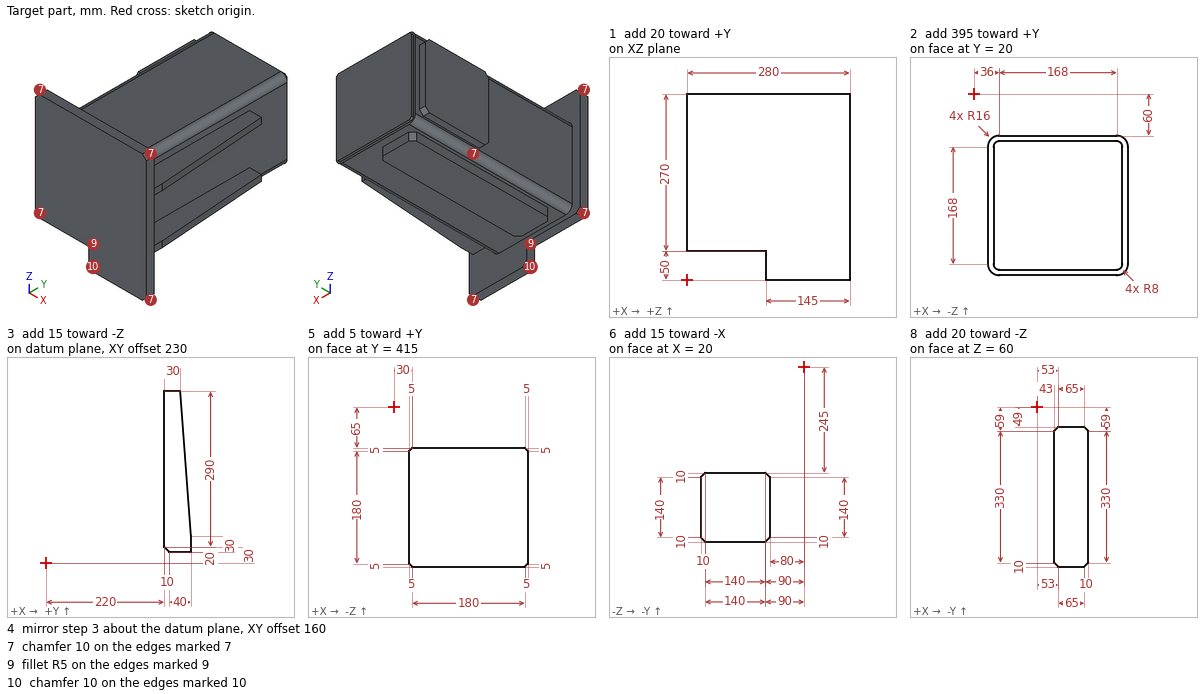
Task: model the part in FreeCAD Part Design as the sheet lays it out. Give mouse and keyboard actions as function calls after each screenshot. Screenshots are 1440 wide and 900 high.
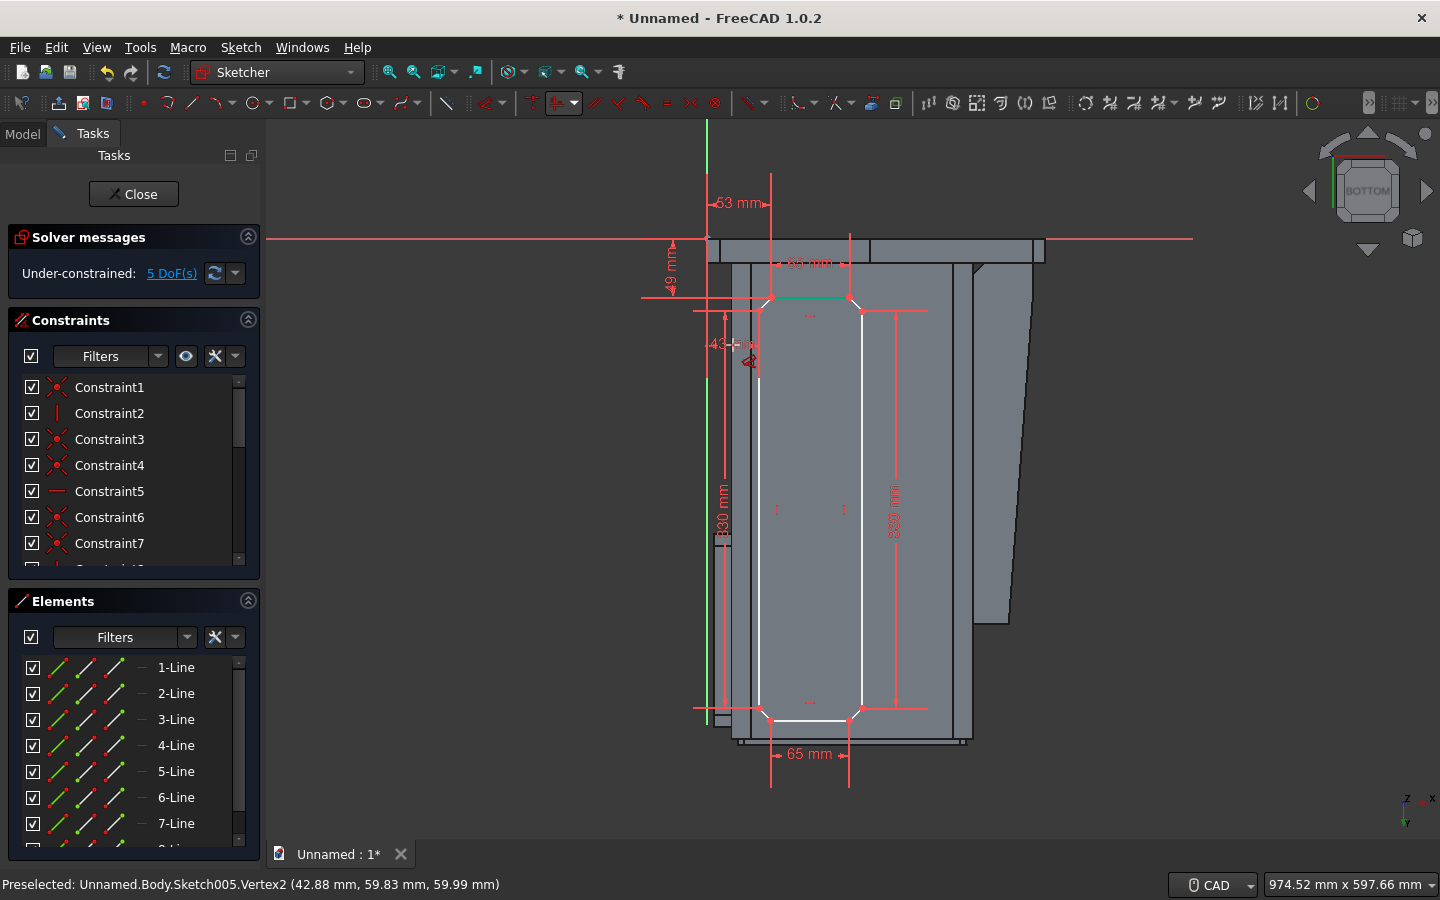
click(759, 311)
click(673, 291)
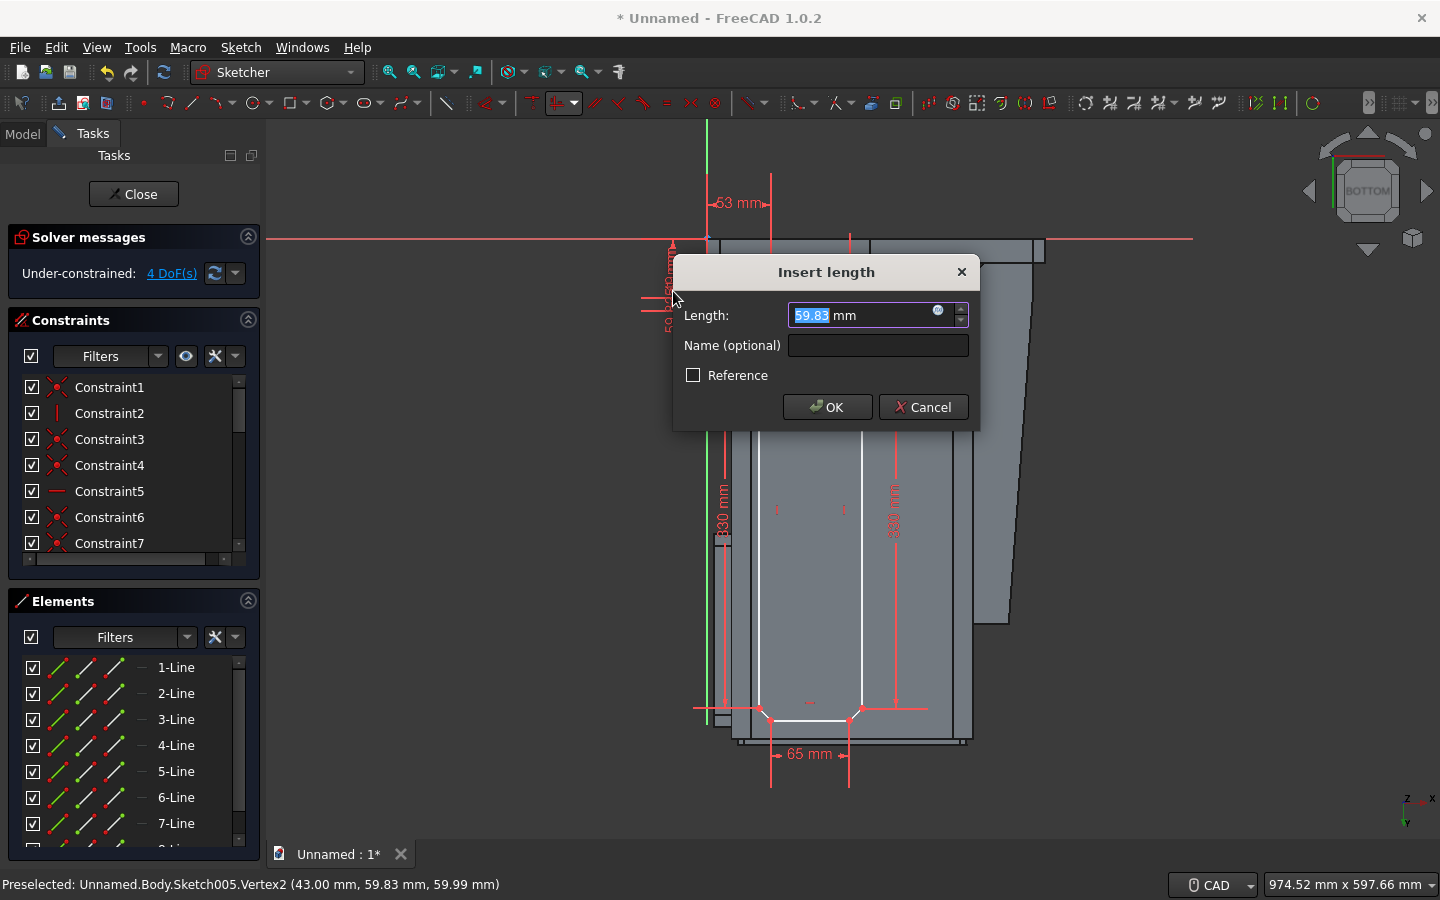
text(59)
key(Return)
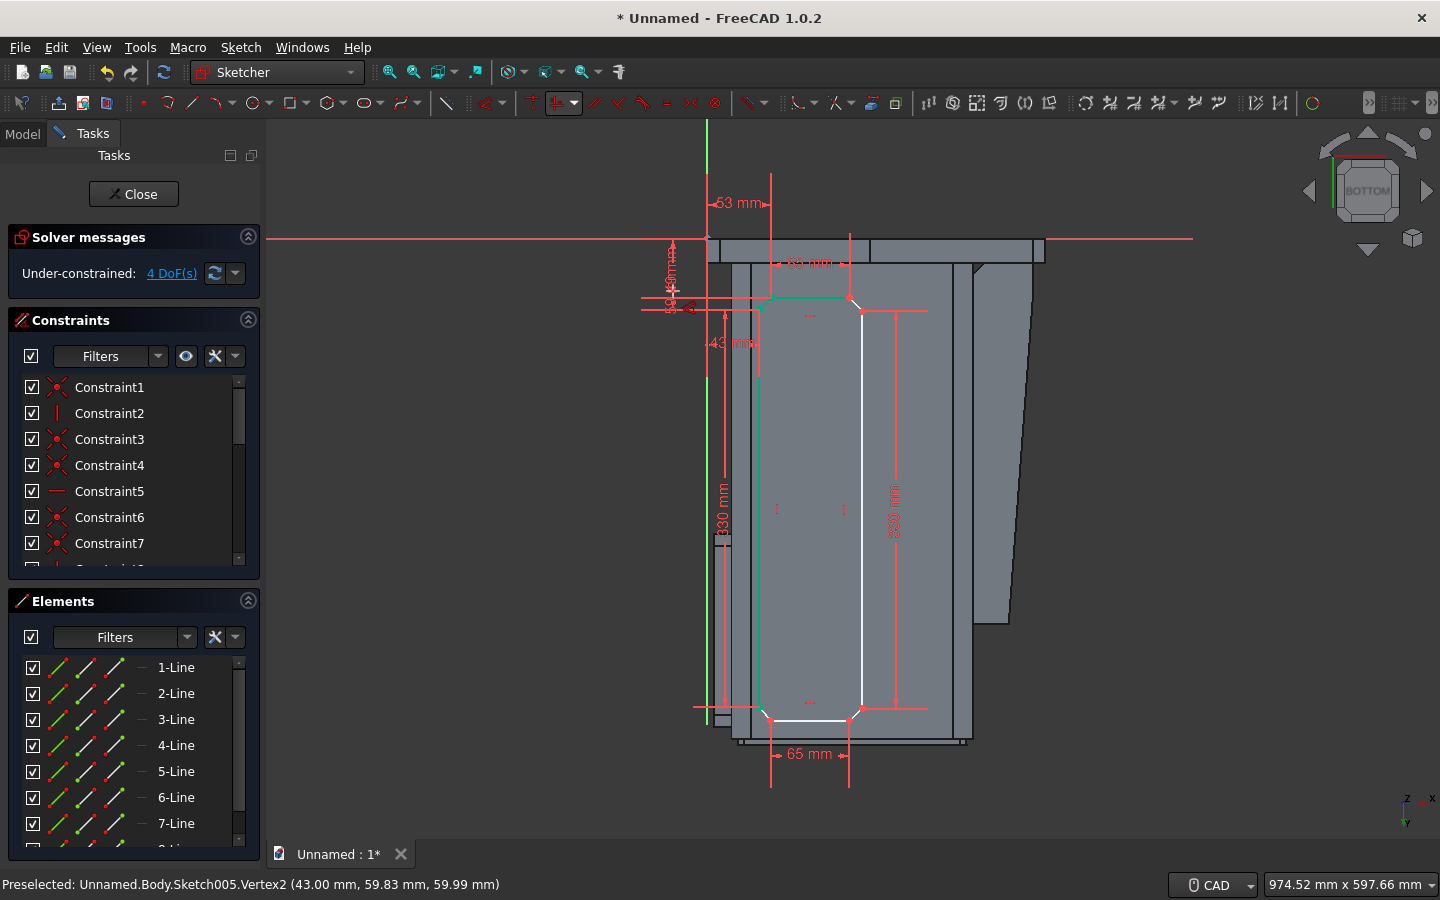
click(771, 721)
click(739, 755)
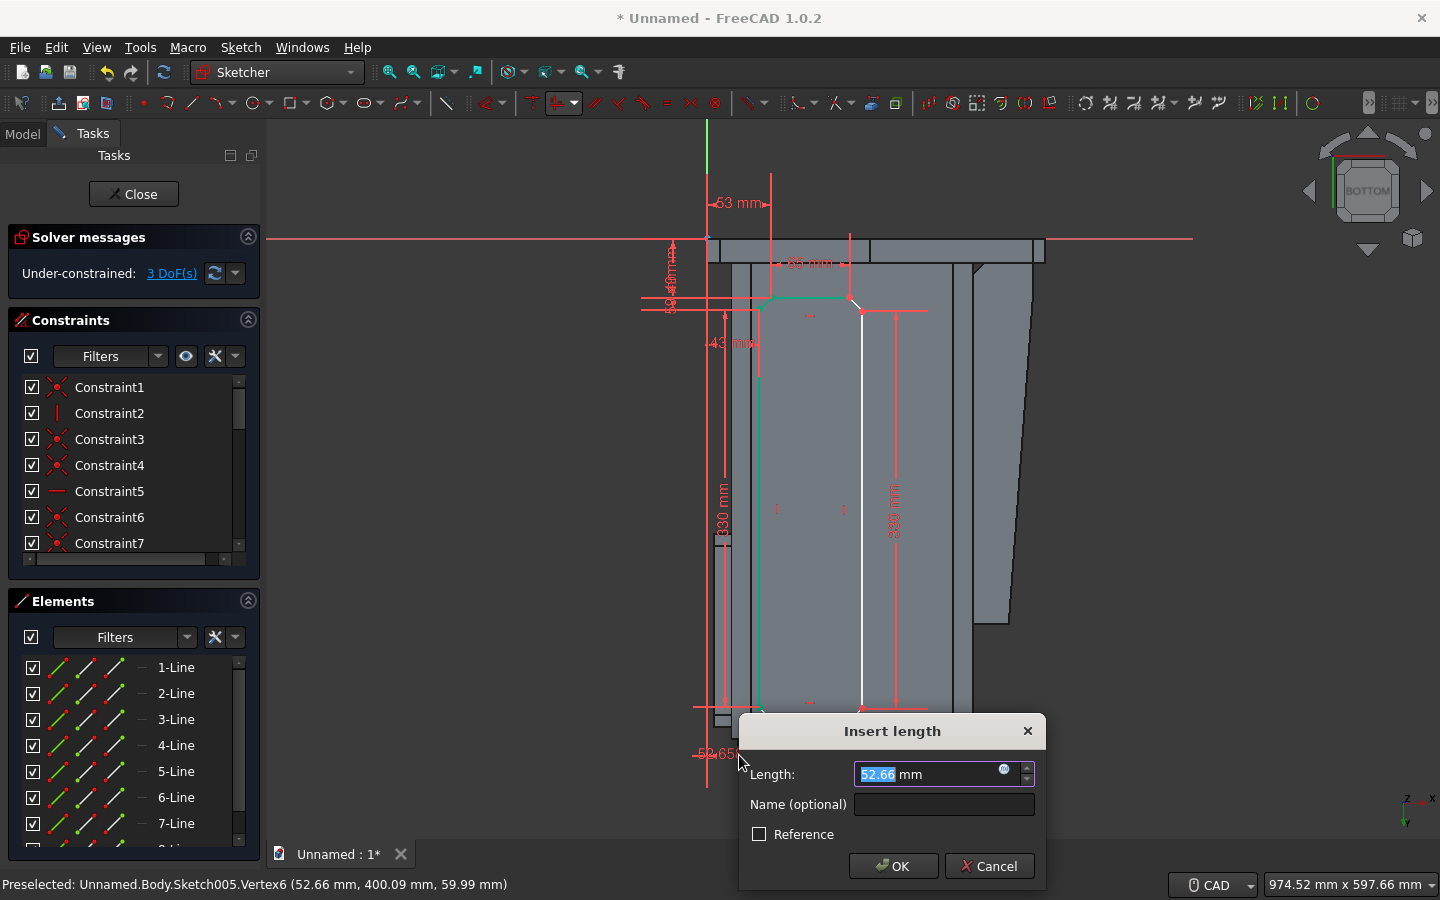
text(53)
key(Return)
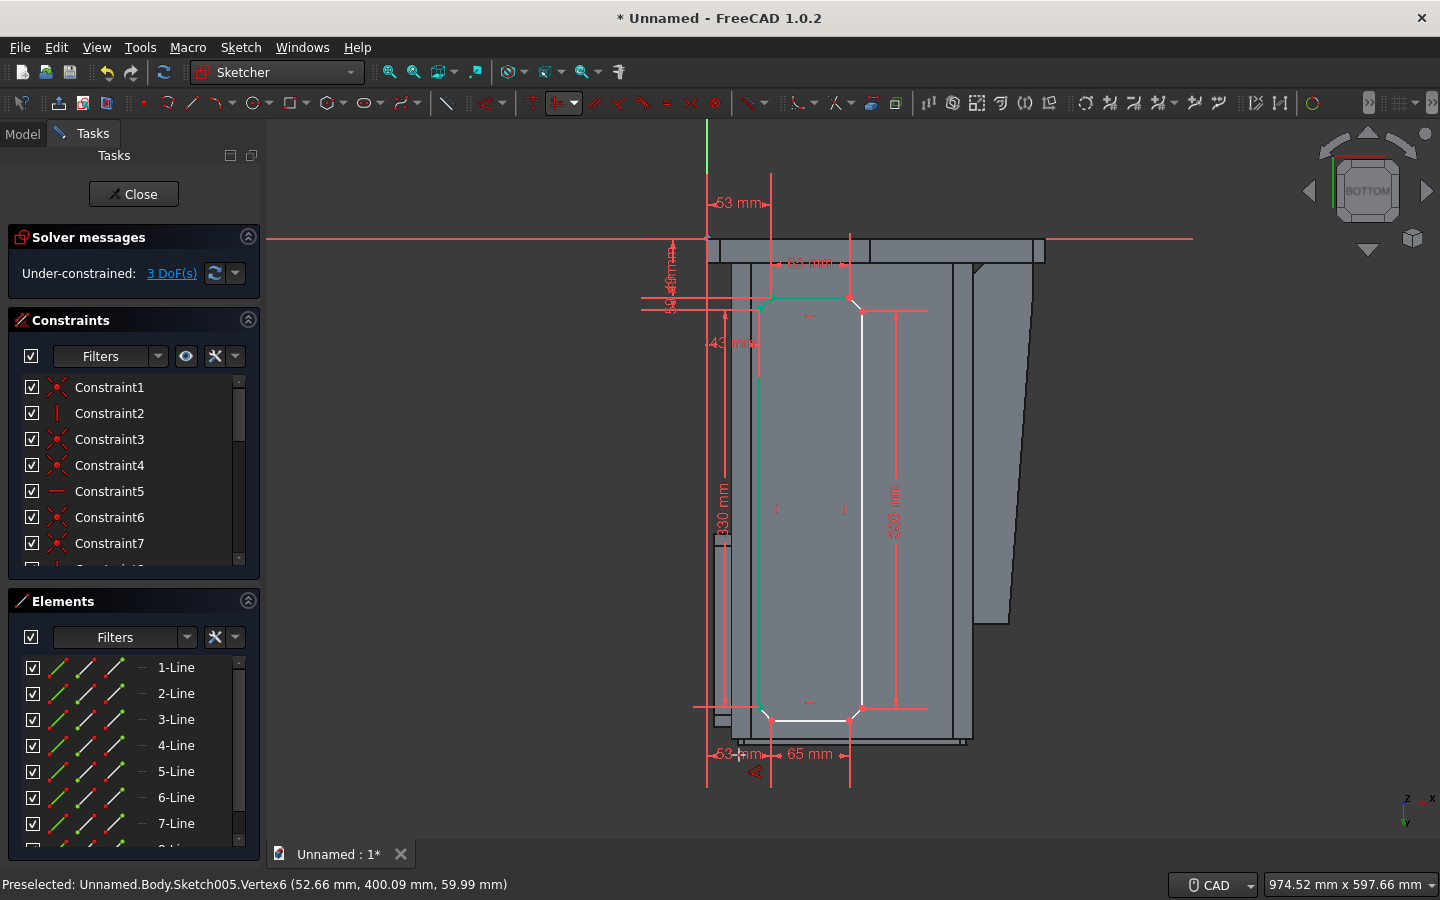
click(862, 311)
click(896, 275)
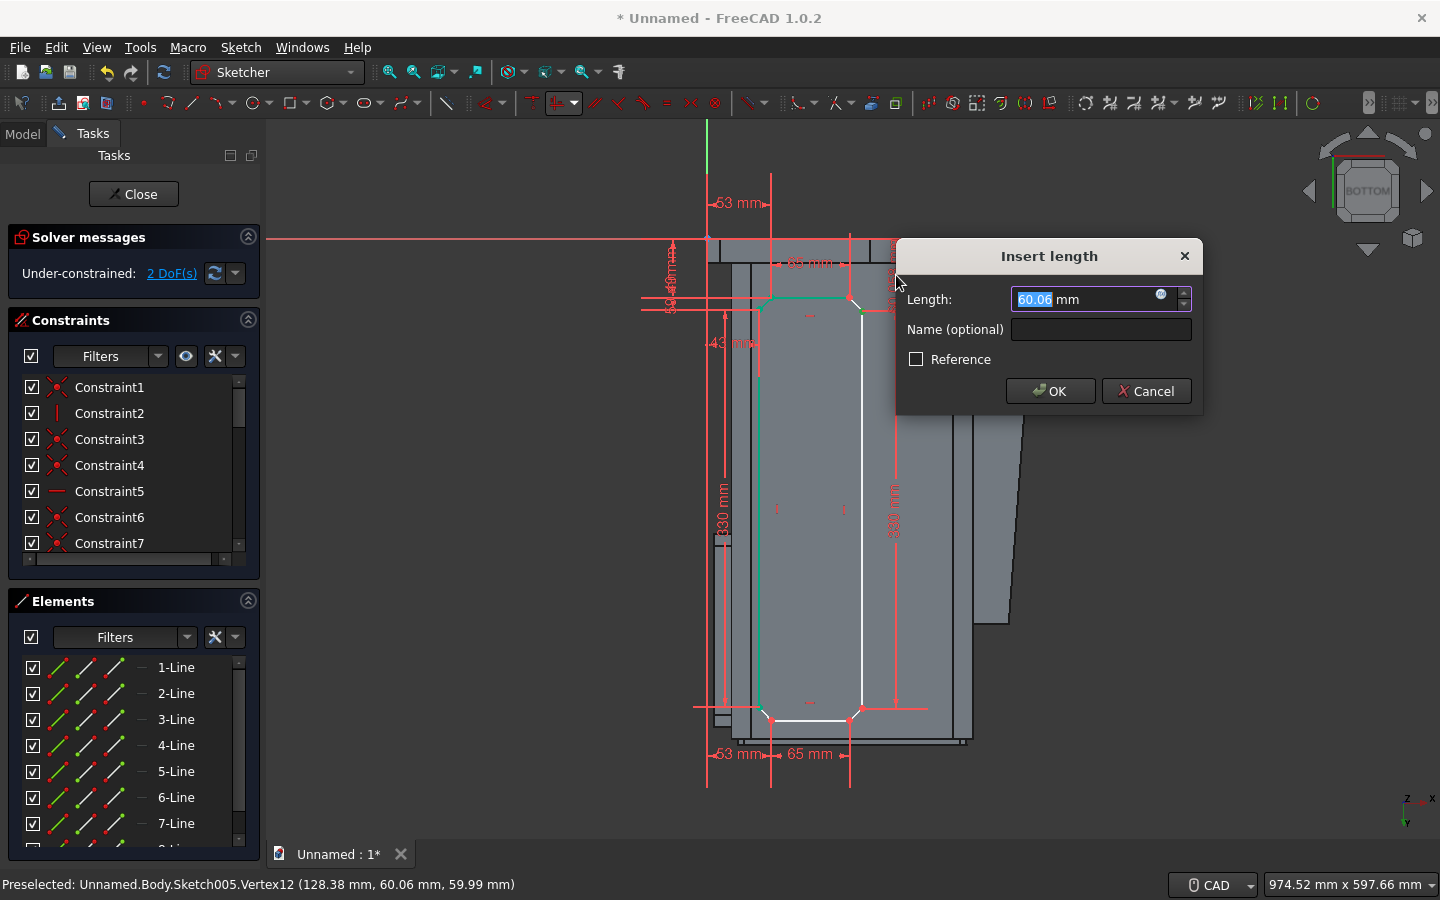
text(59)
key(Return)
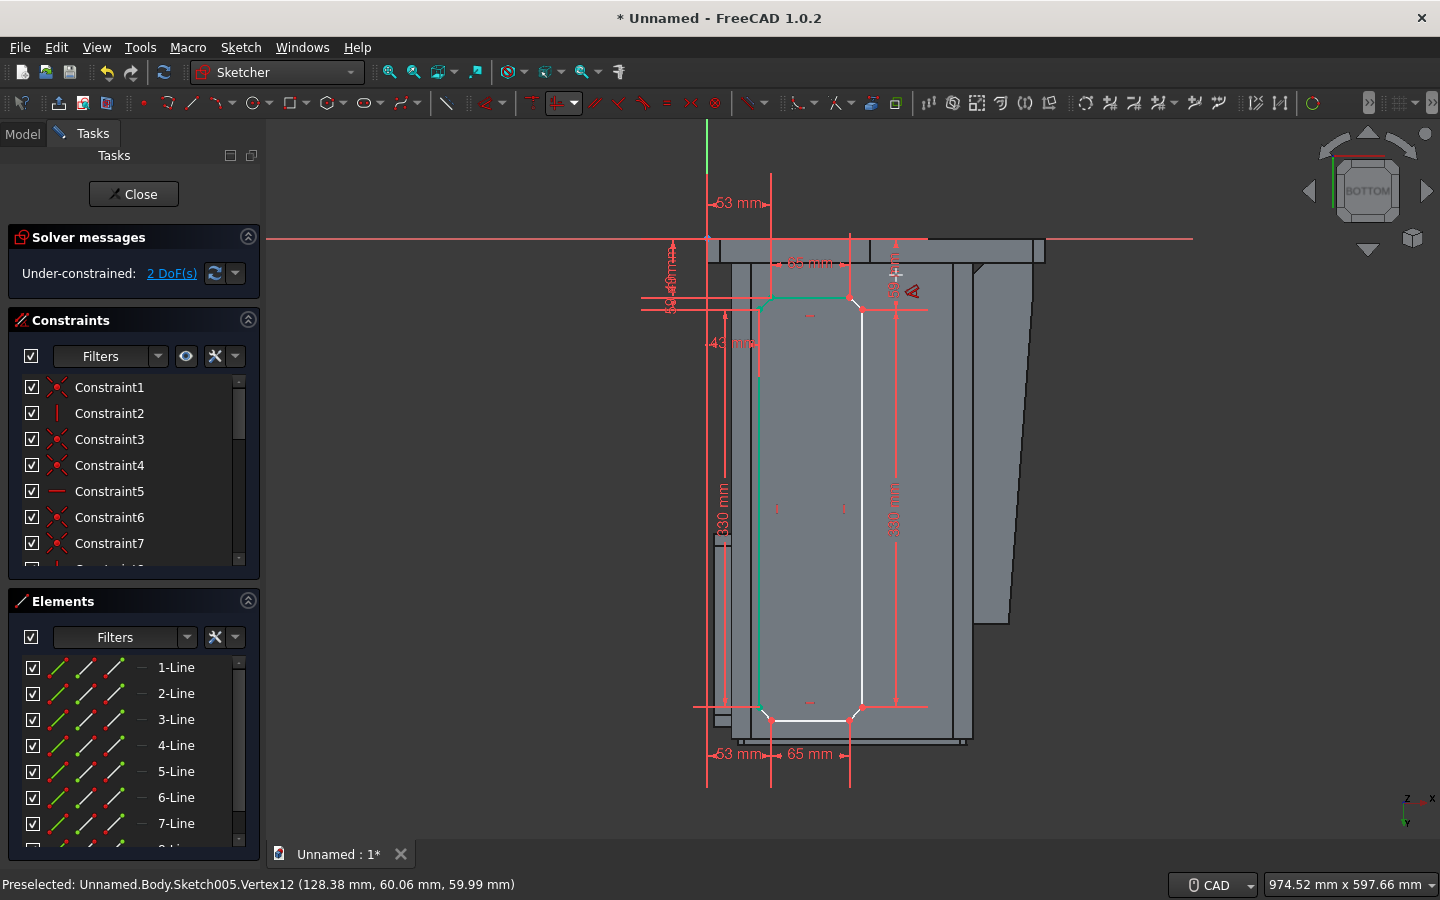
scroll(765, 714, up, 6)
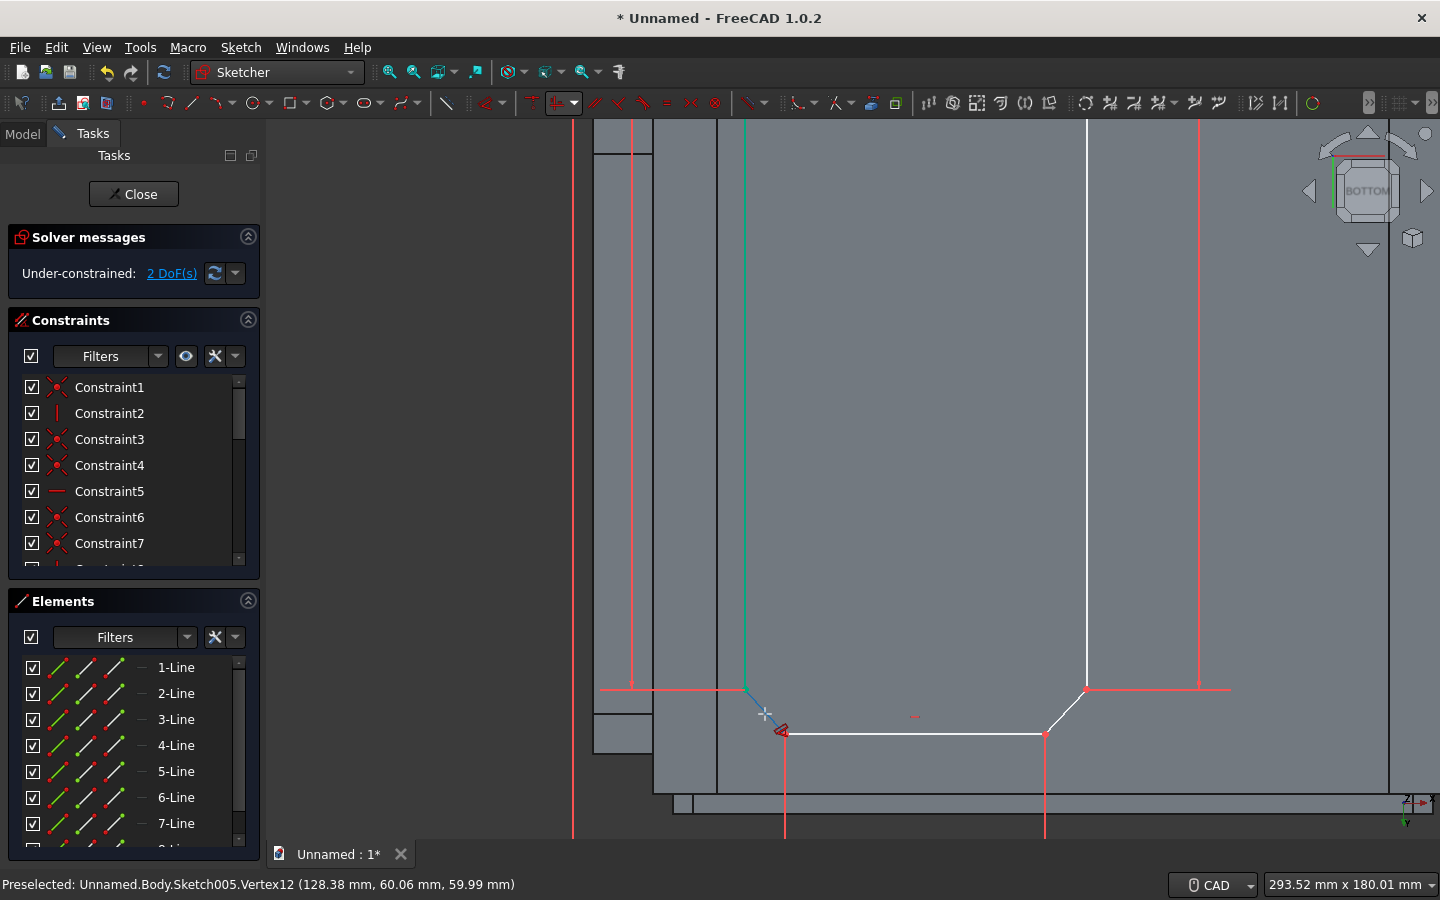
click(765, 712)
click(711, 712)